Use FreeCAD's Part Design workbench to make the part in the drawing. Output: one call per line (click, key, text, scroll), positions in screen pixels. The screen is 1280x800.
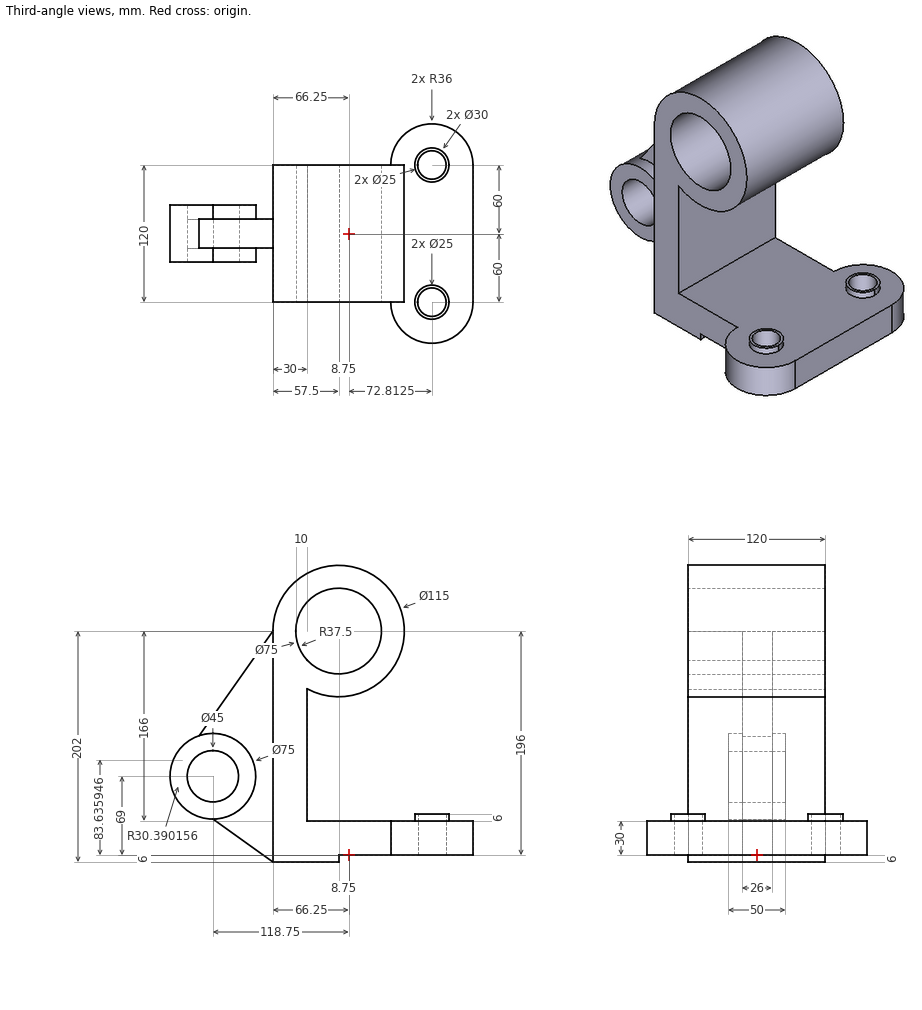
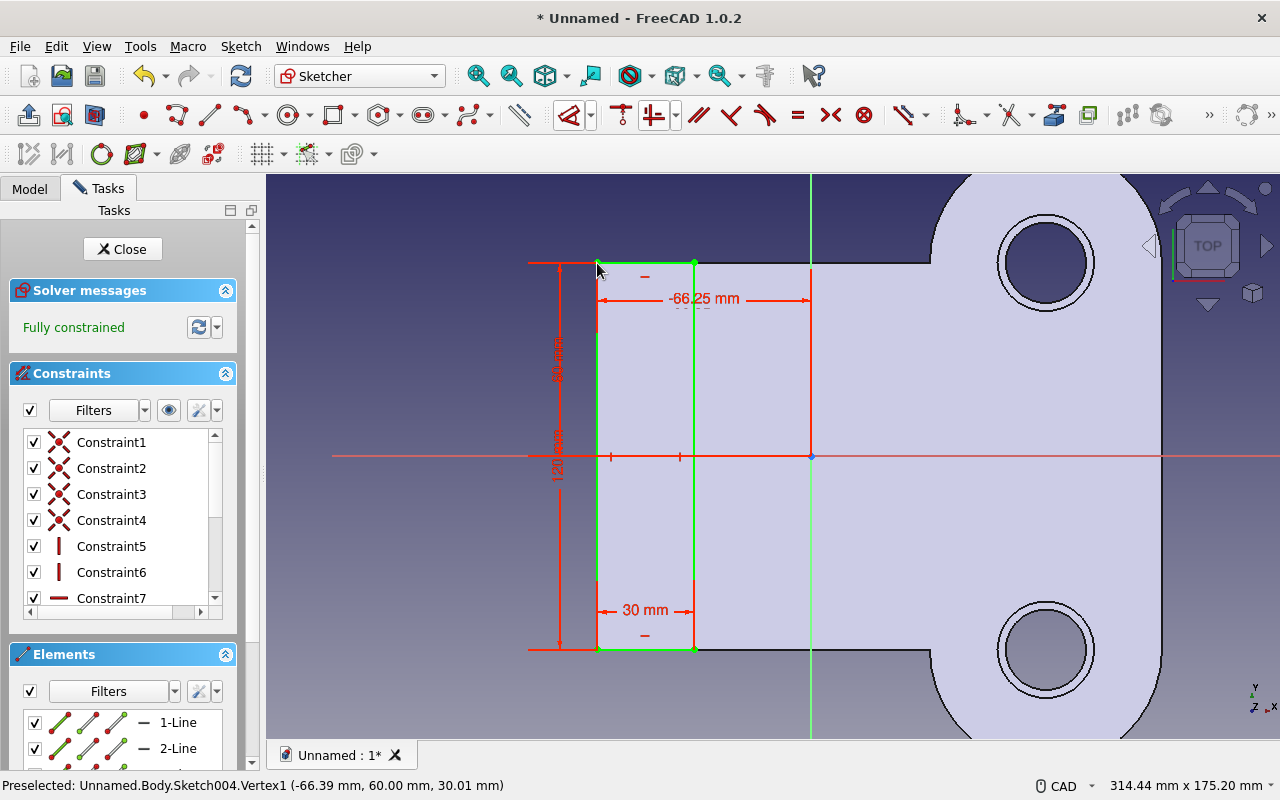
click(123, 249)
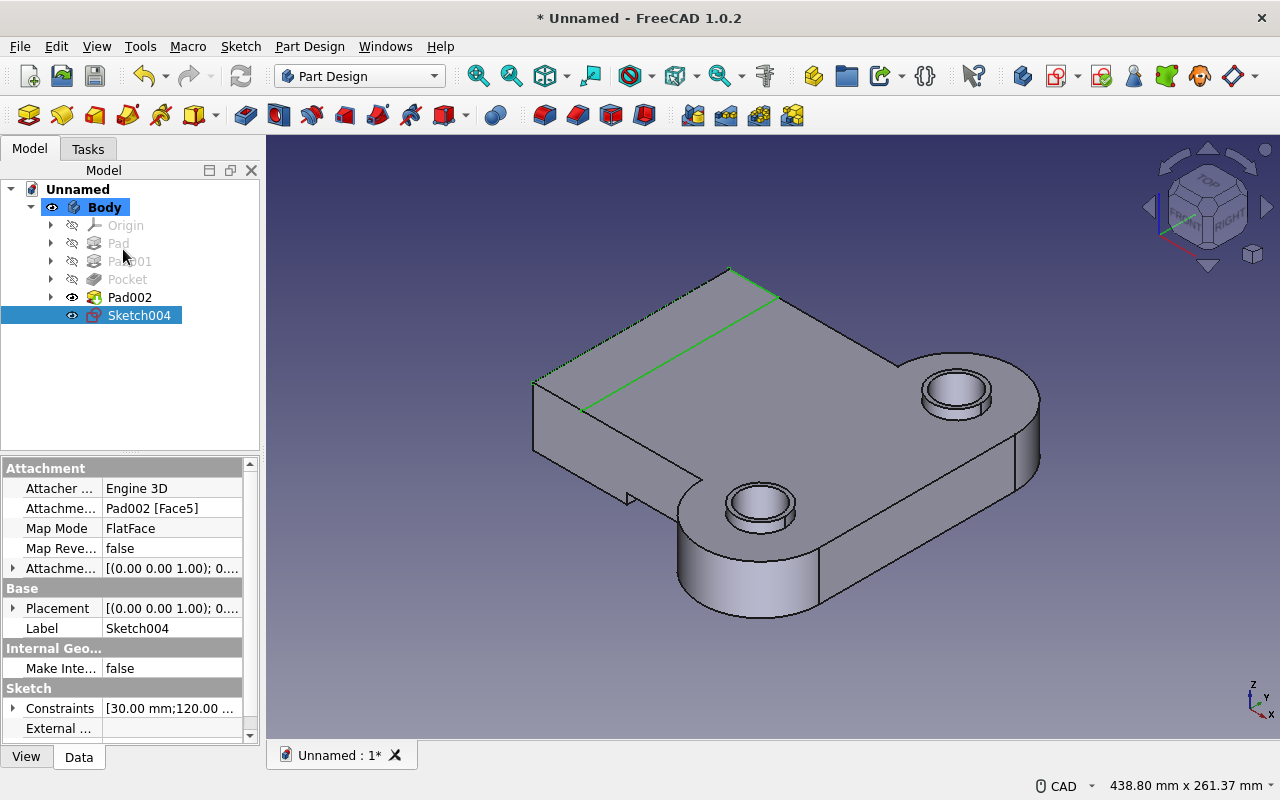
click(29, 116)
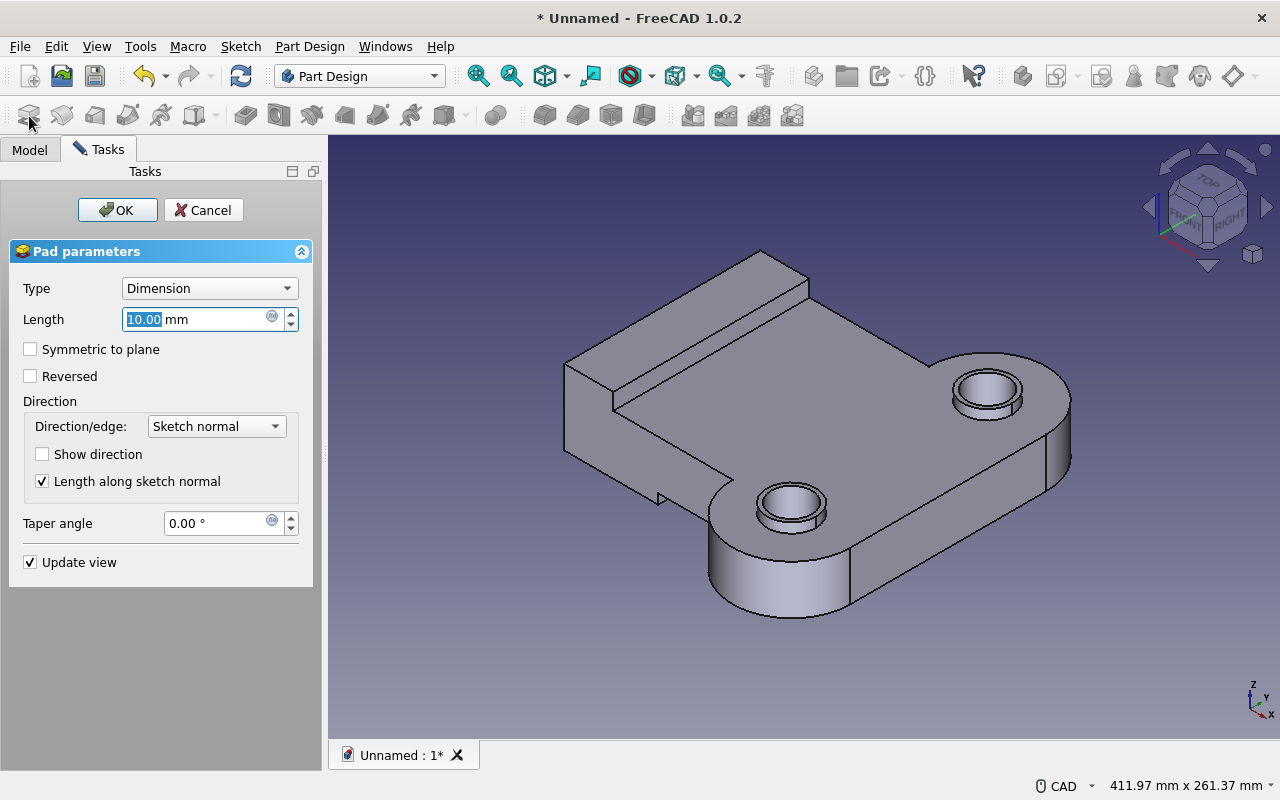
text(166)
key(Tab)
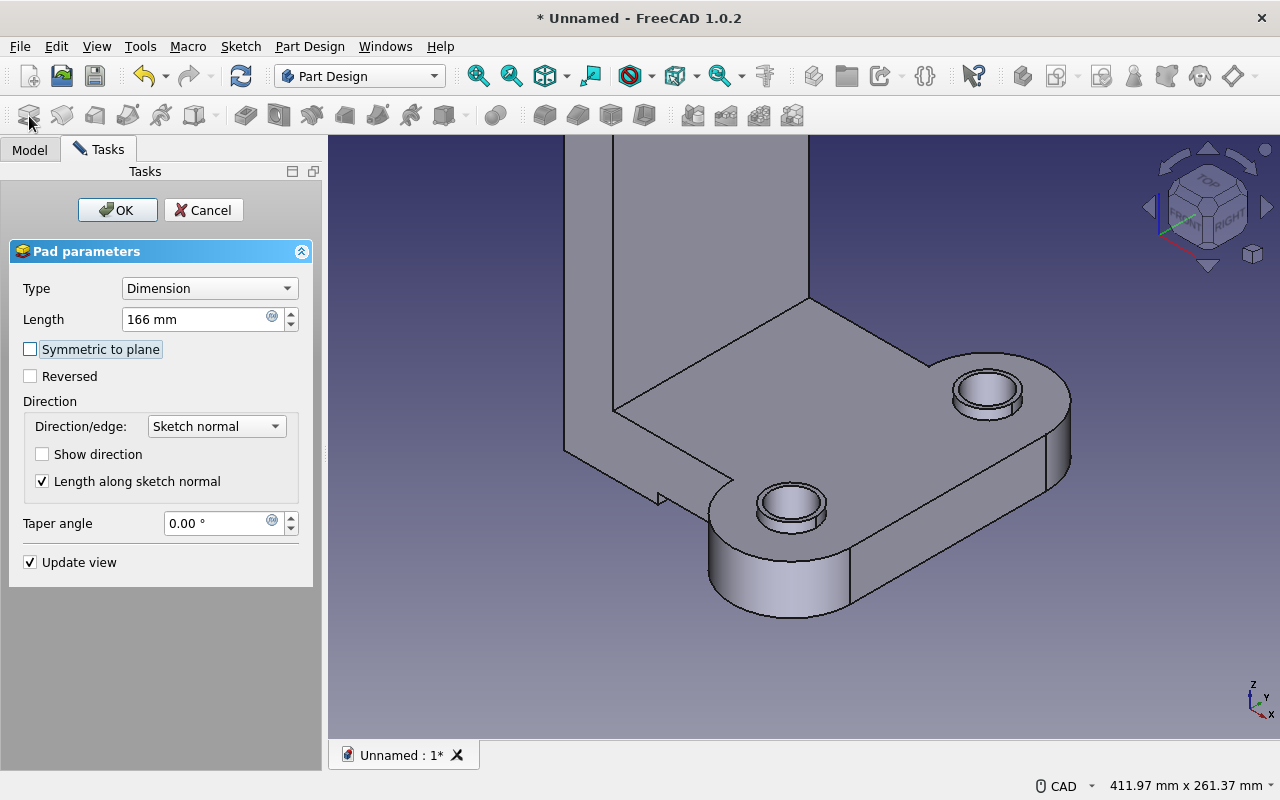
click(118, 210)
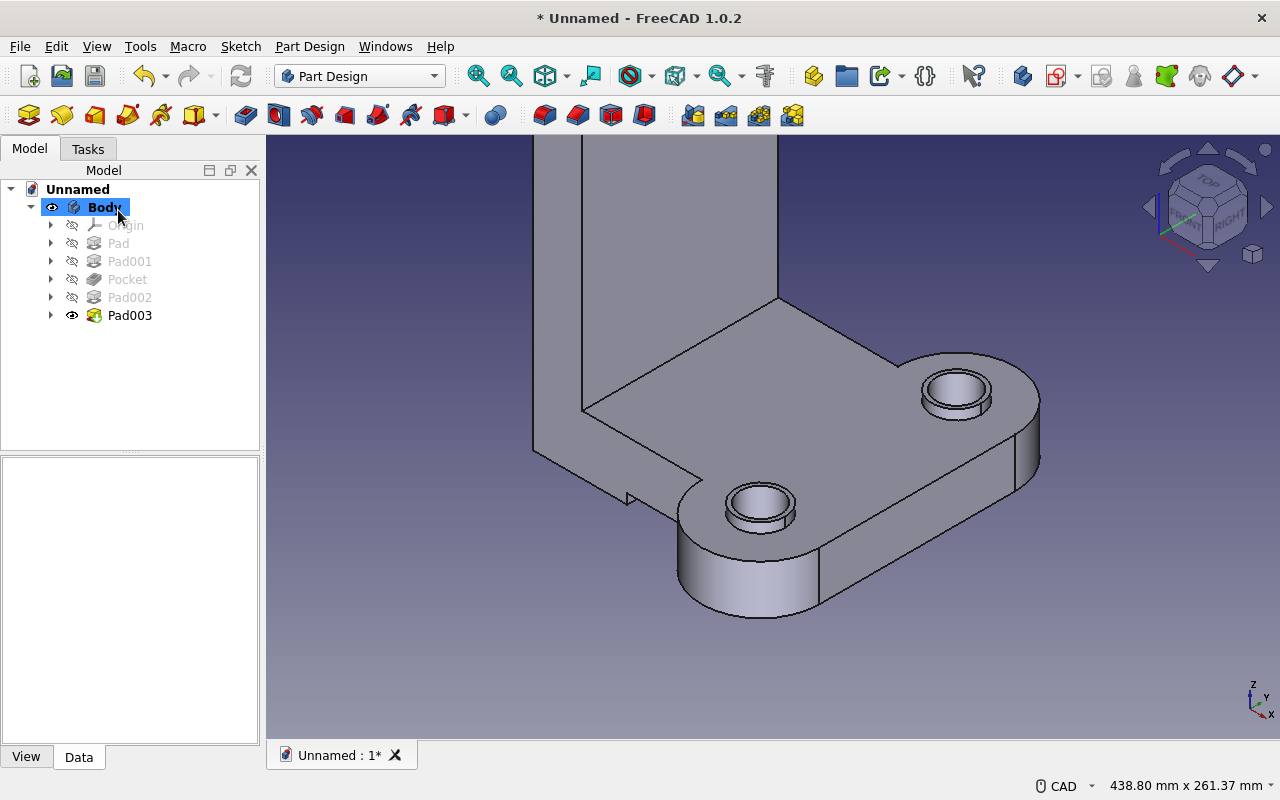
click(479, 76)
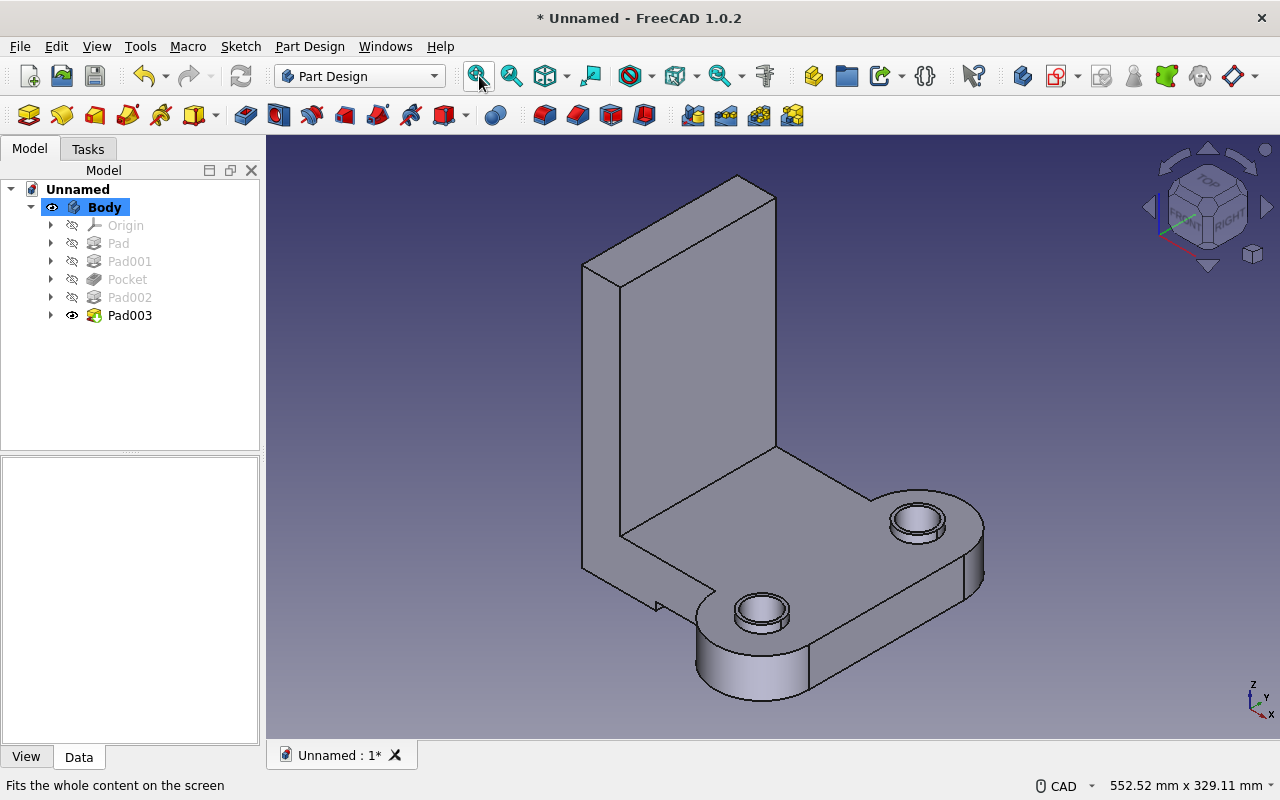
click(1056, 76)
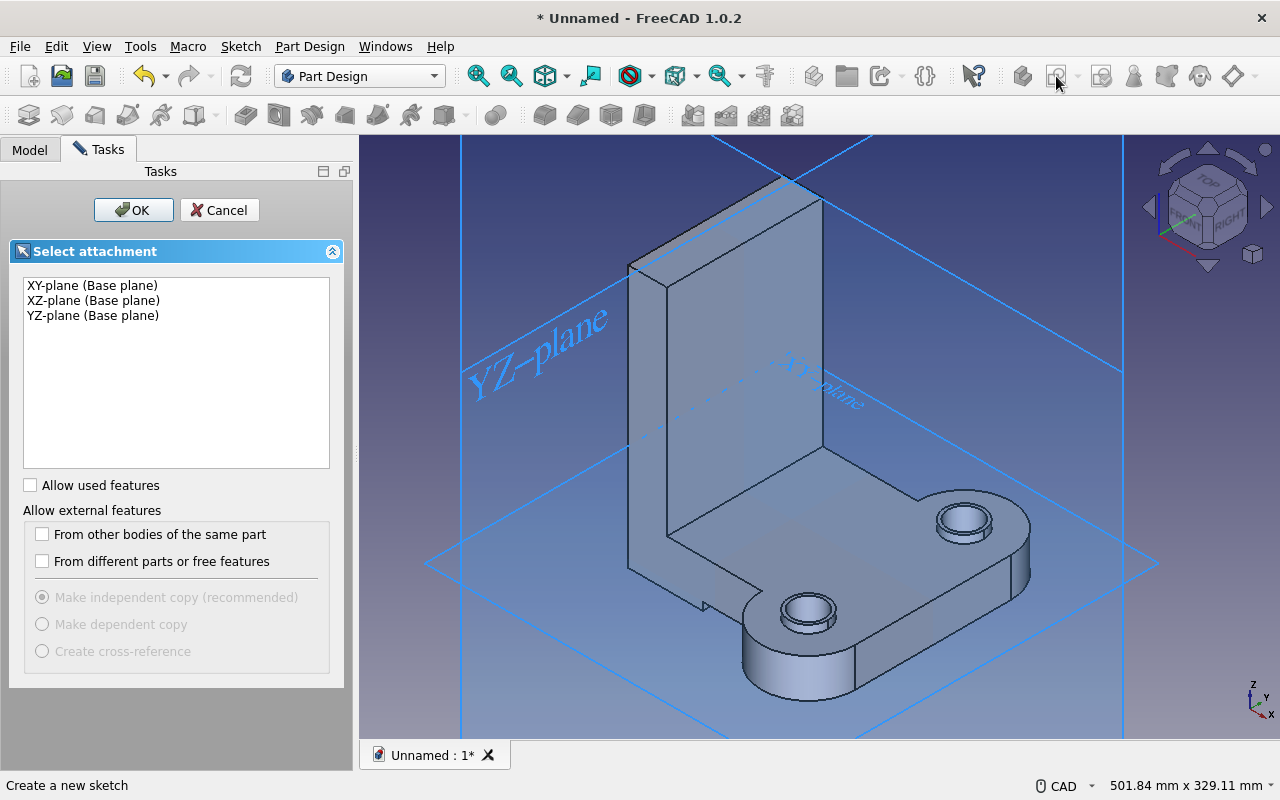
click(84, 300)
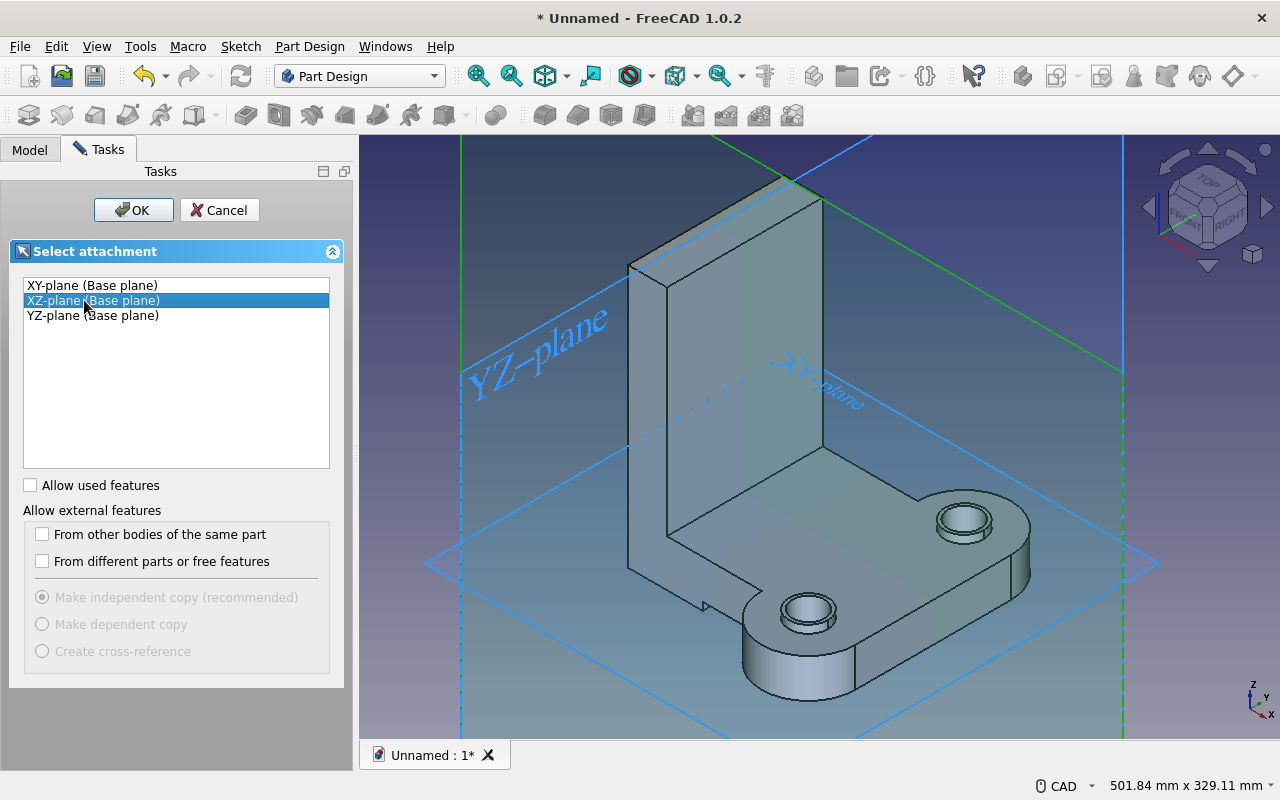
click(134, 210)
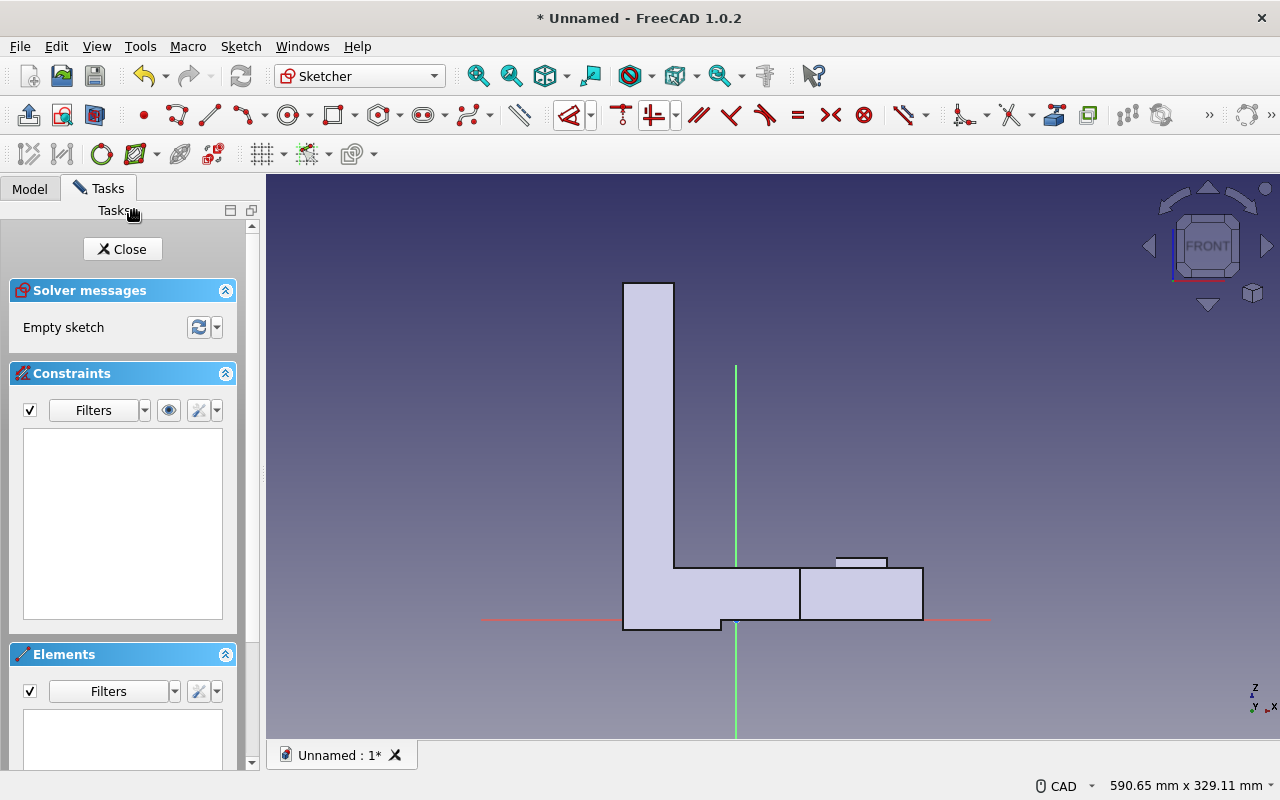
key(q)
key(s)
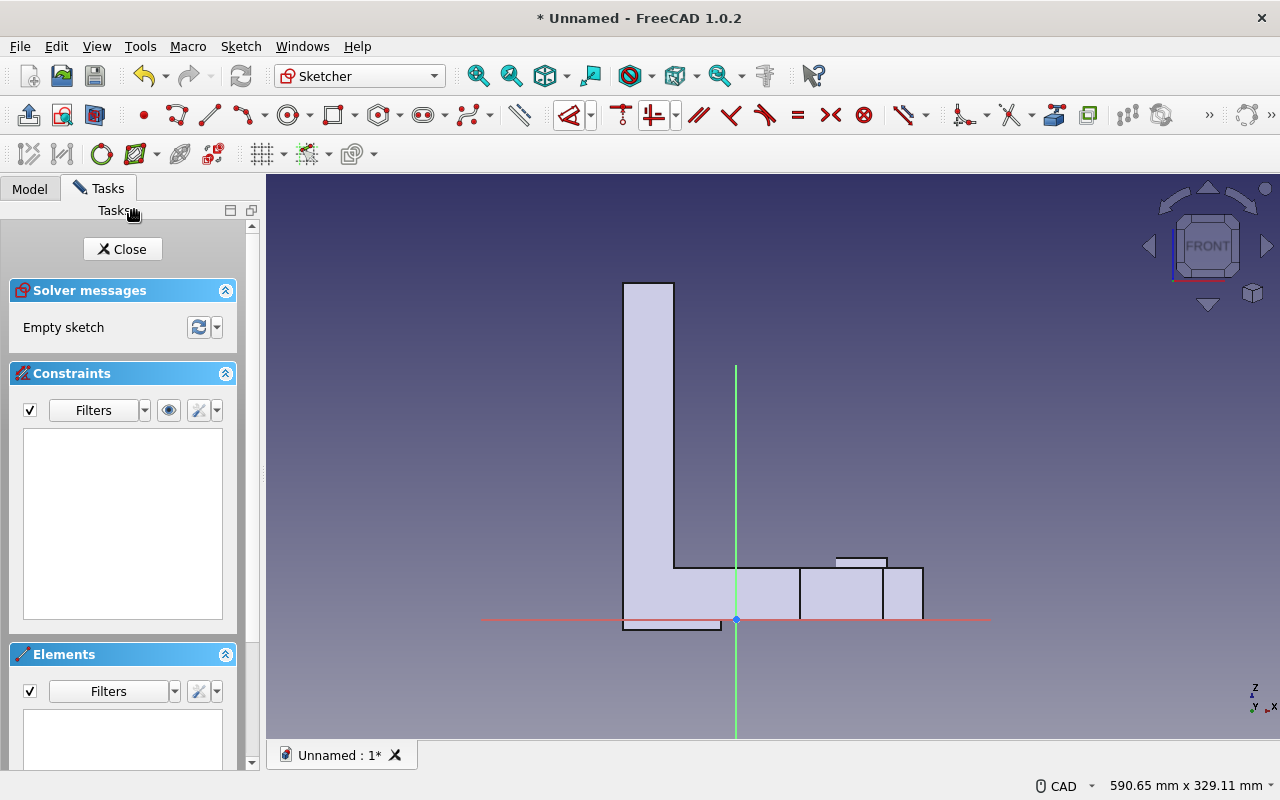
scroll(628, 703, down, 1)